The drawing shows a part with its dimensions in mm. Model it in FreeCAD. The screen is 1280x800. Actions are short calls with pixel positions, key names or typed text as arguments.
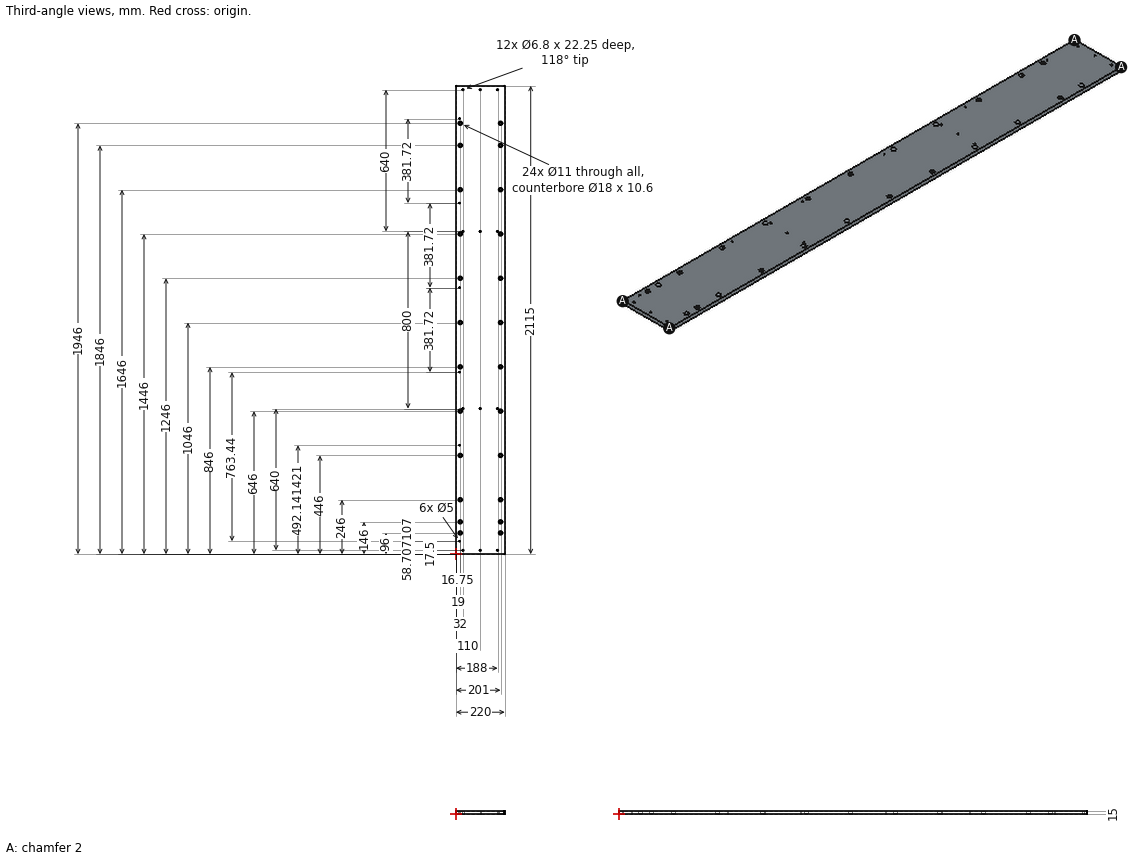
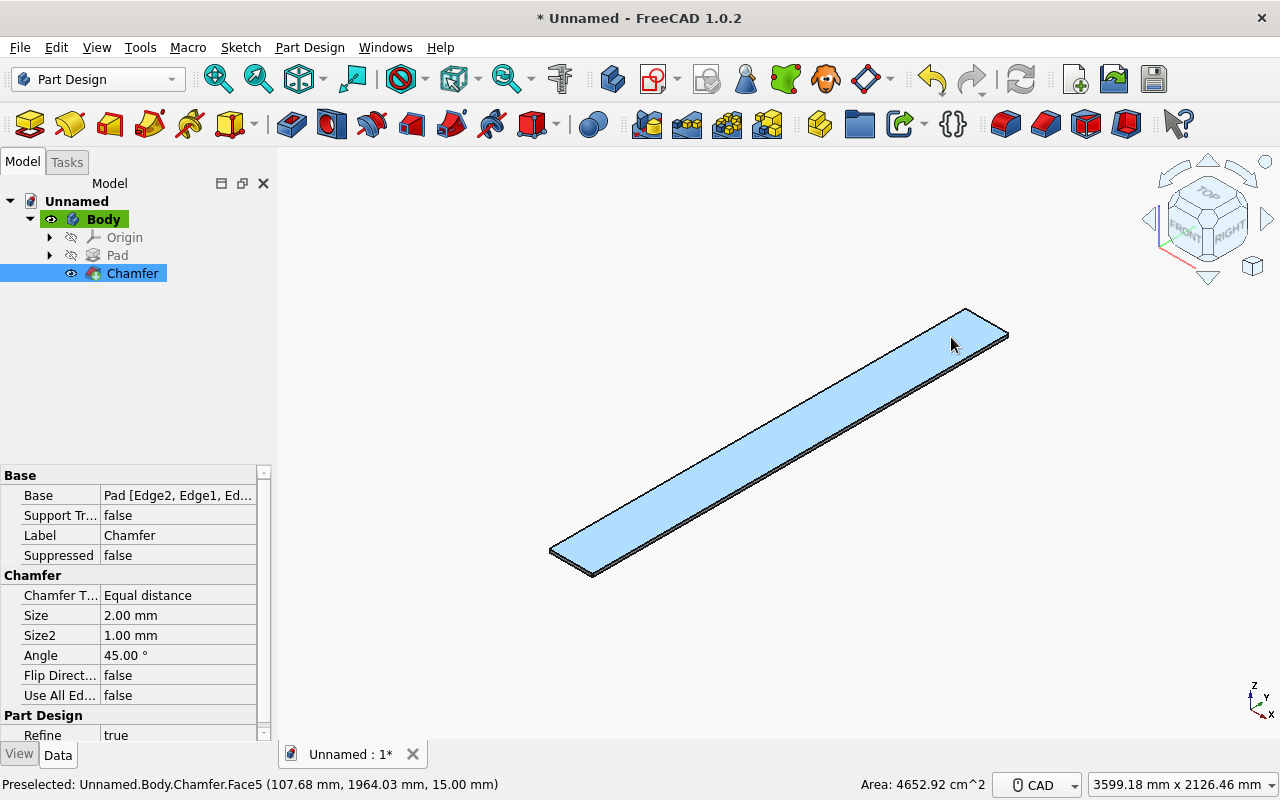
click(654, 80)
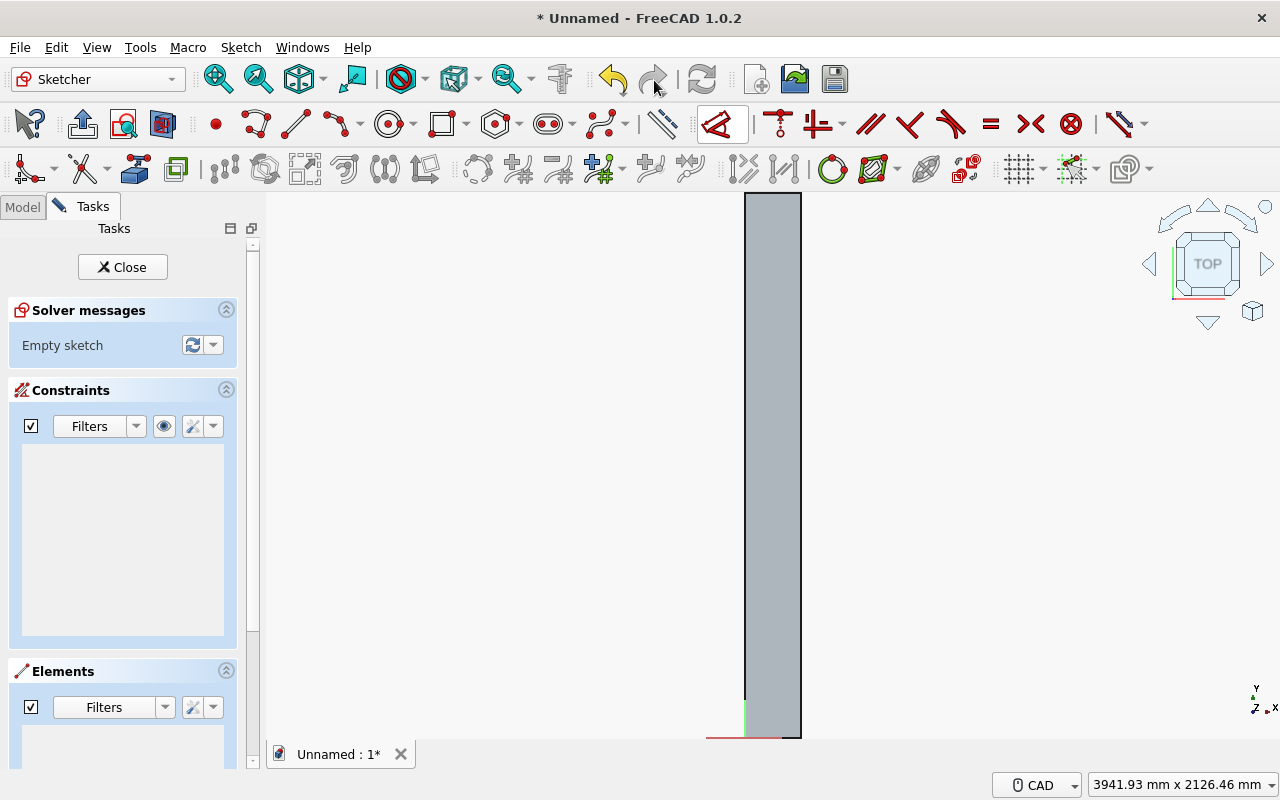
scroll(573, 462, down, 2)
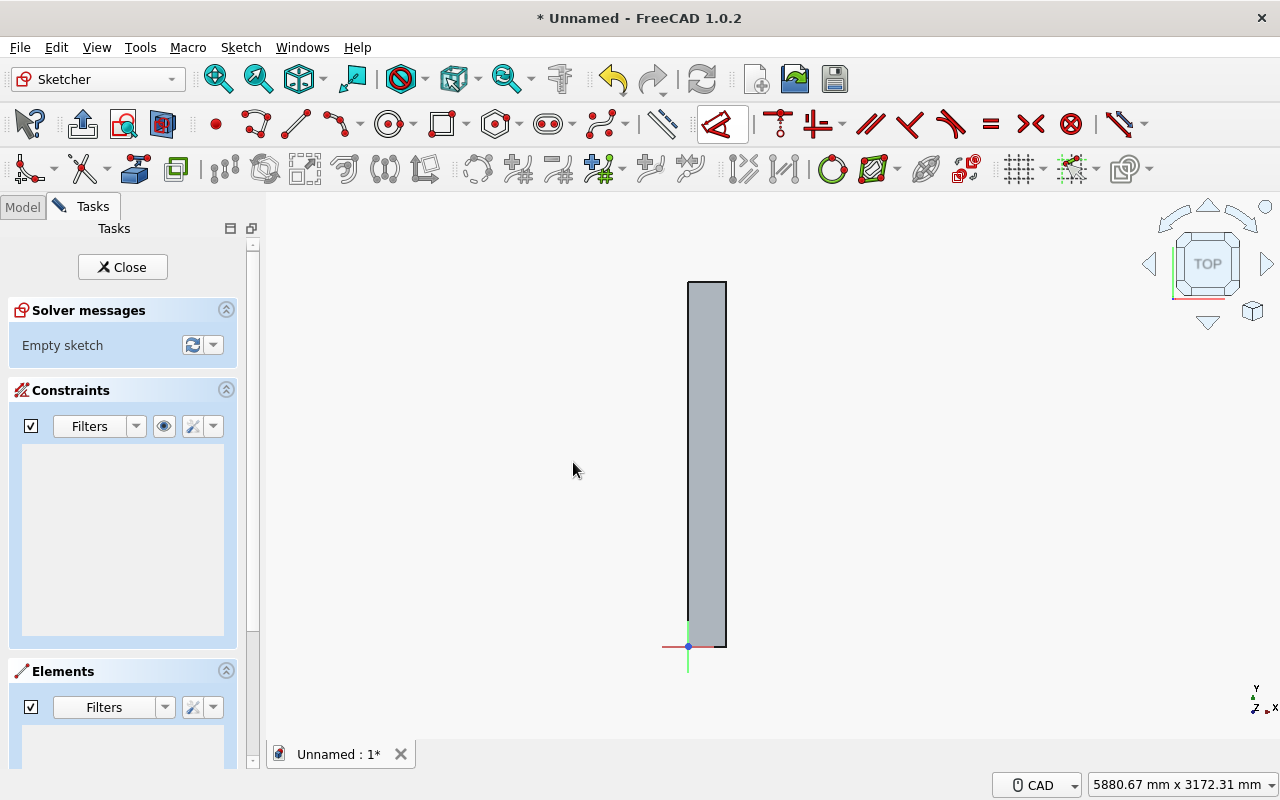
click(390, 124)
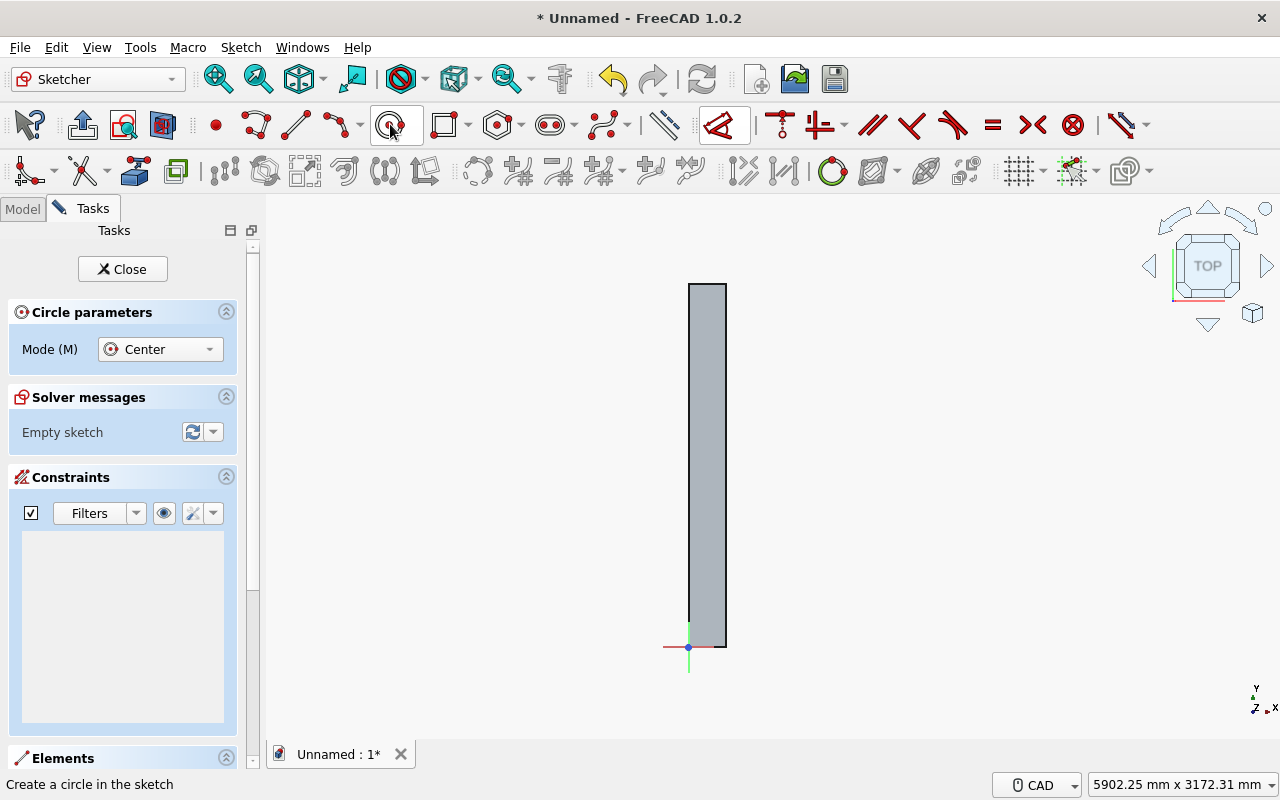
scroll(694, 287, up, 19)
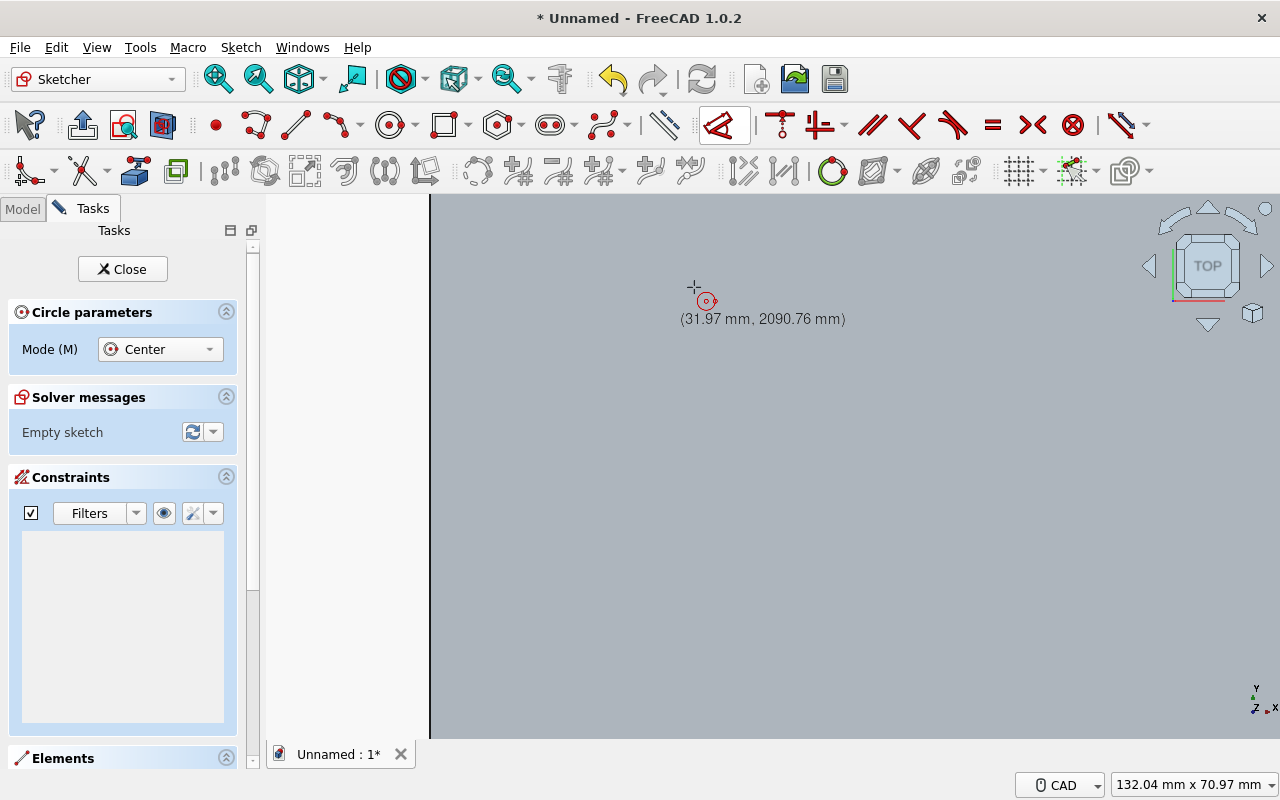
scroll(704, 466, down, 15)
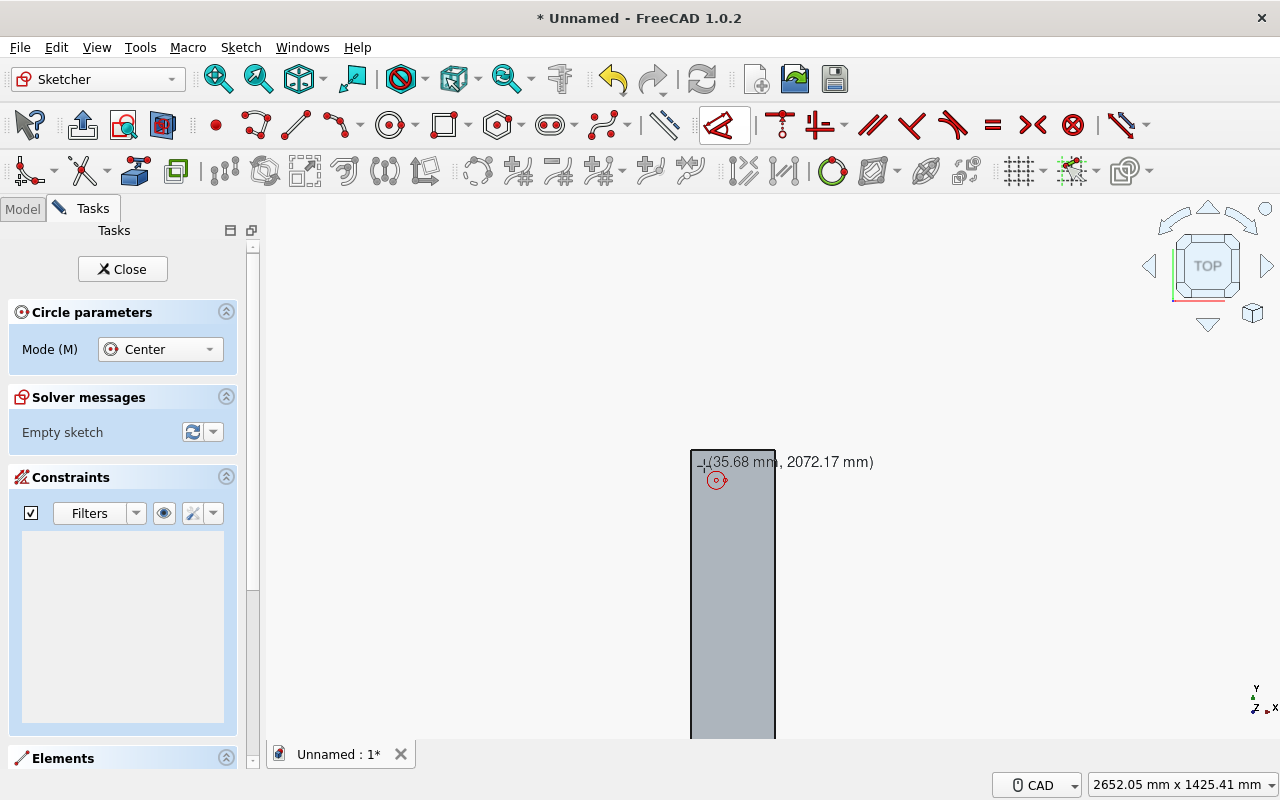
scroll(691, 239, down, 5)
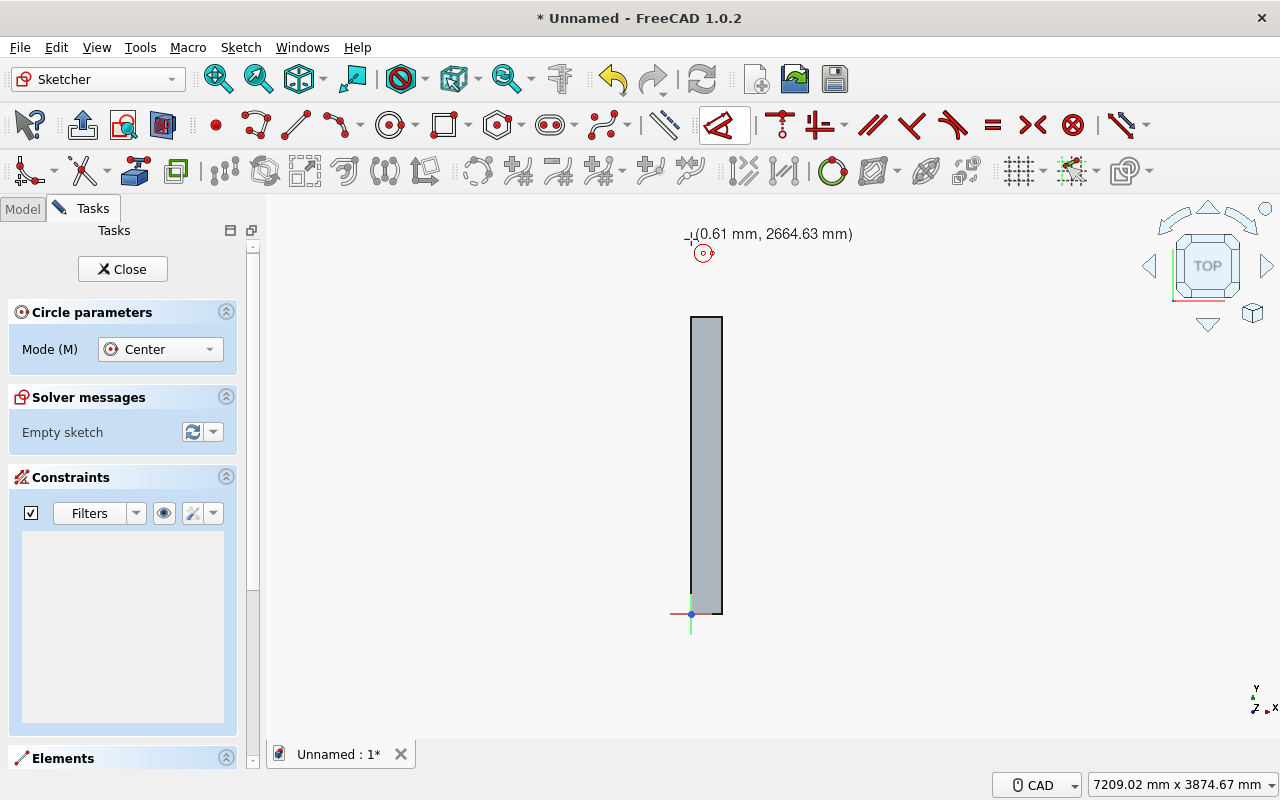
scroll(696, 319, up, 7)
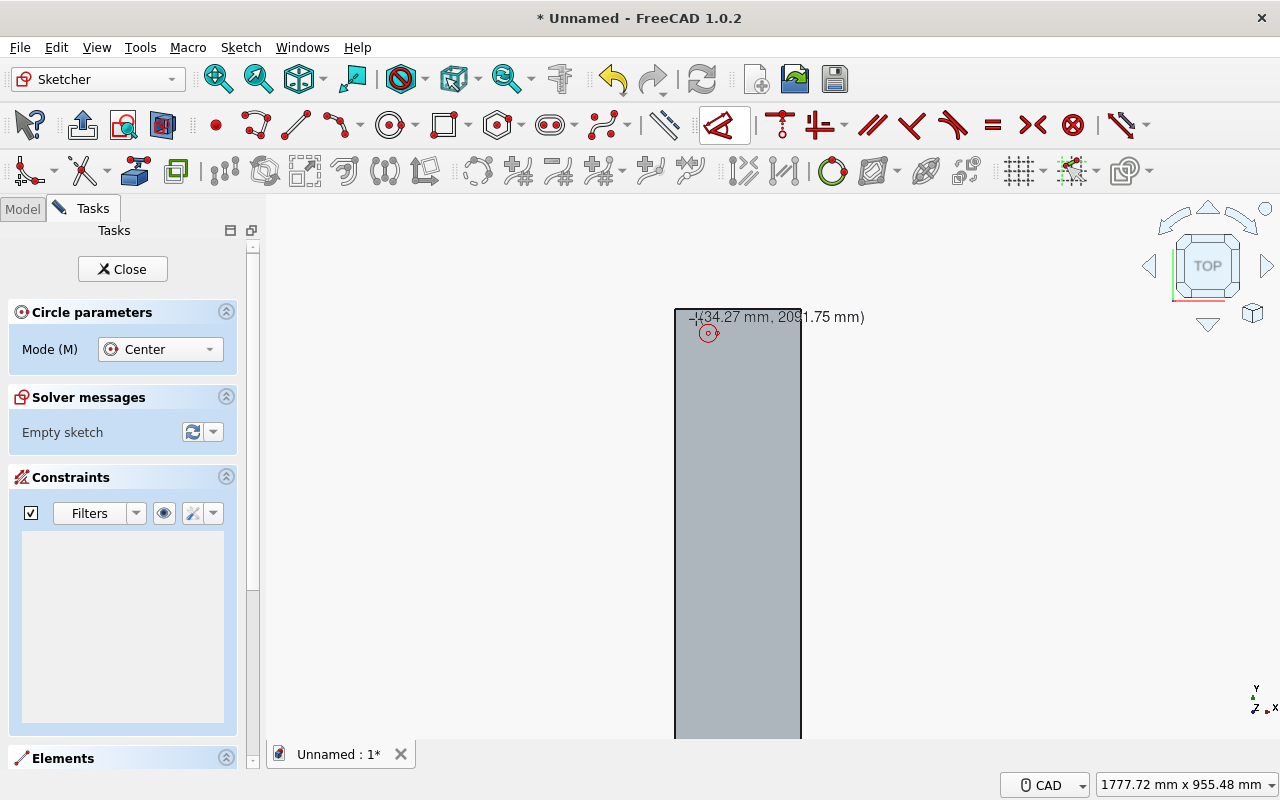
click(693, 319)
move(695, 318)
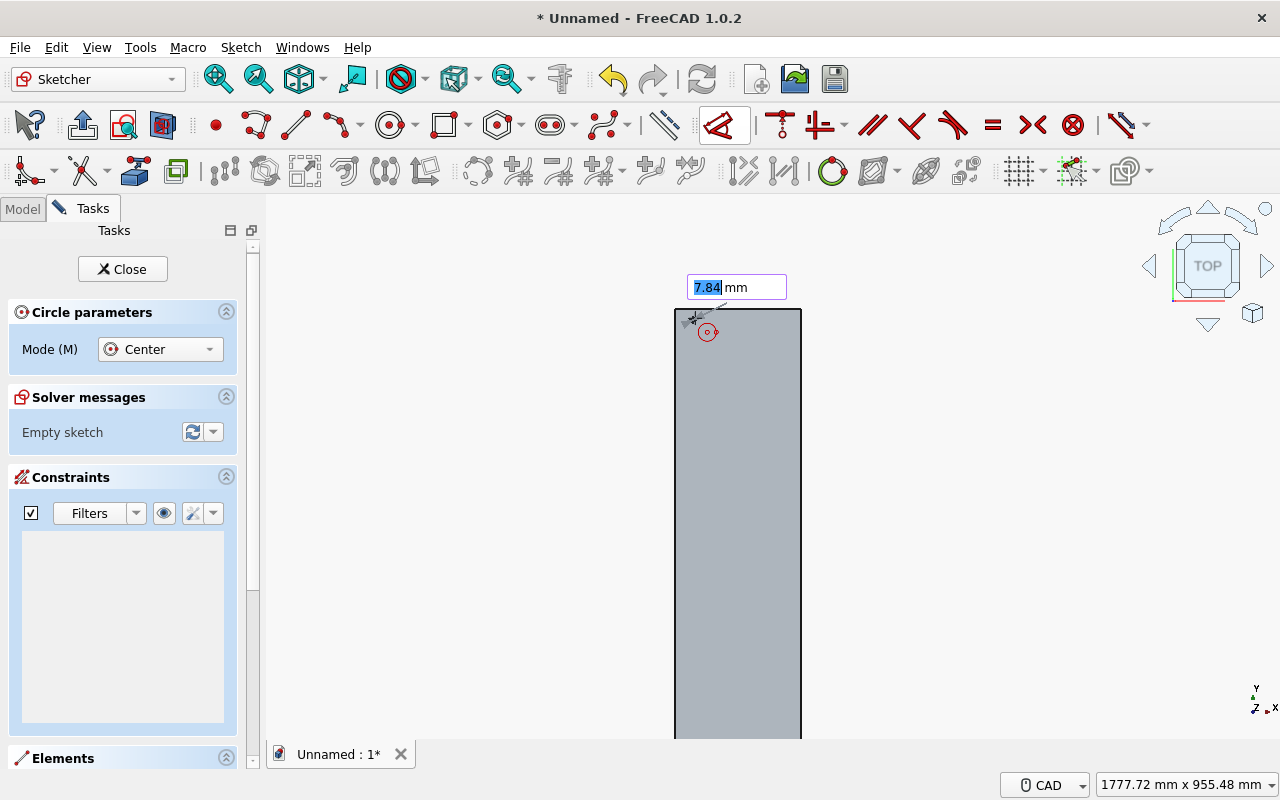
text(6.8)
key(Return)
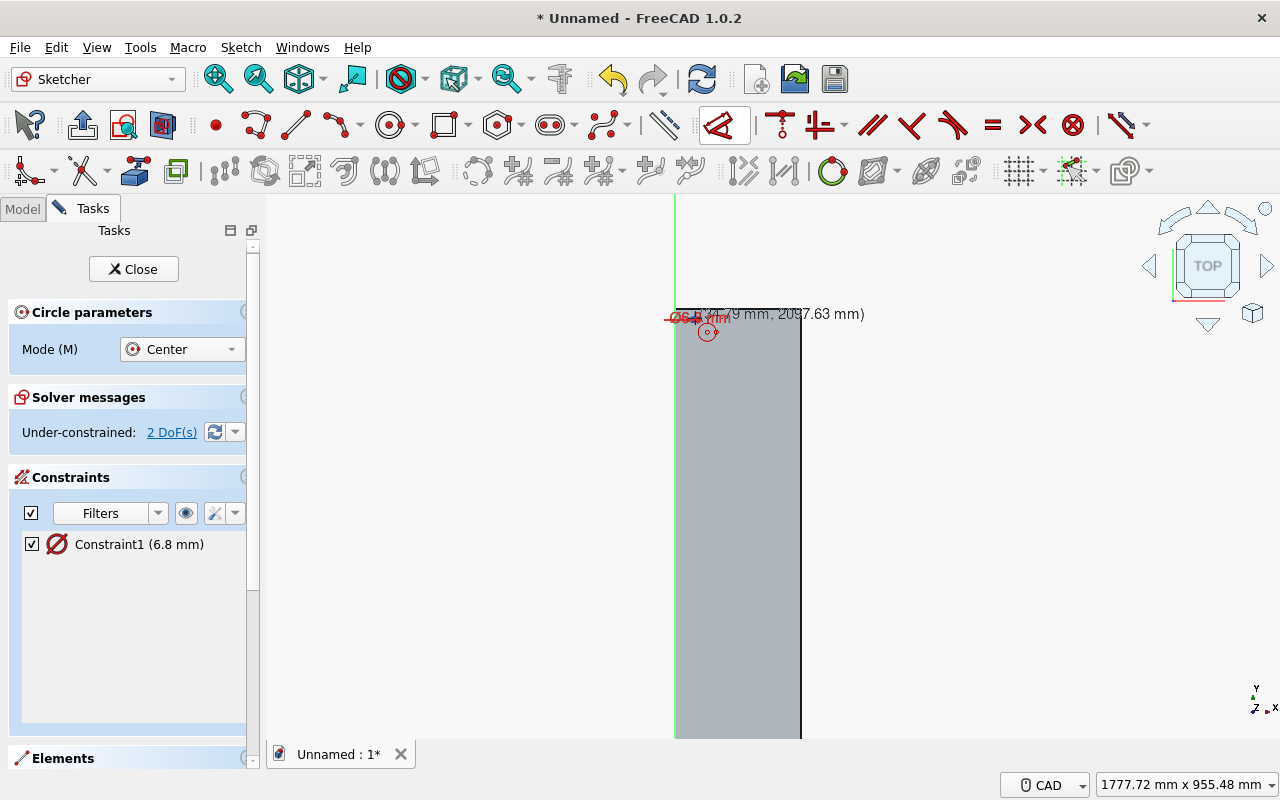
scroll(693, 684, up, 13)